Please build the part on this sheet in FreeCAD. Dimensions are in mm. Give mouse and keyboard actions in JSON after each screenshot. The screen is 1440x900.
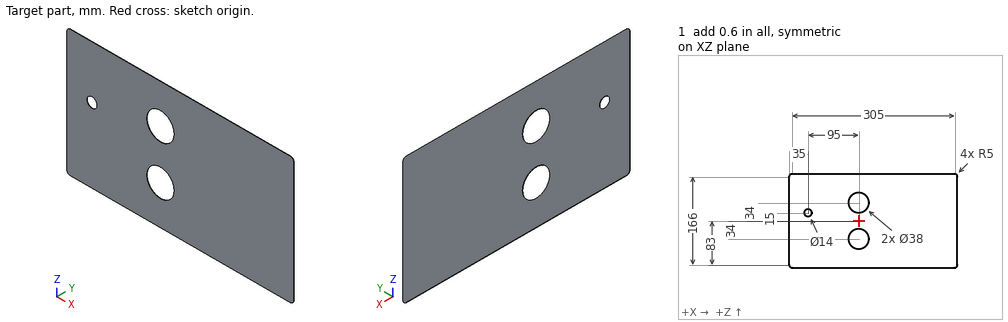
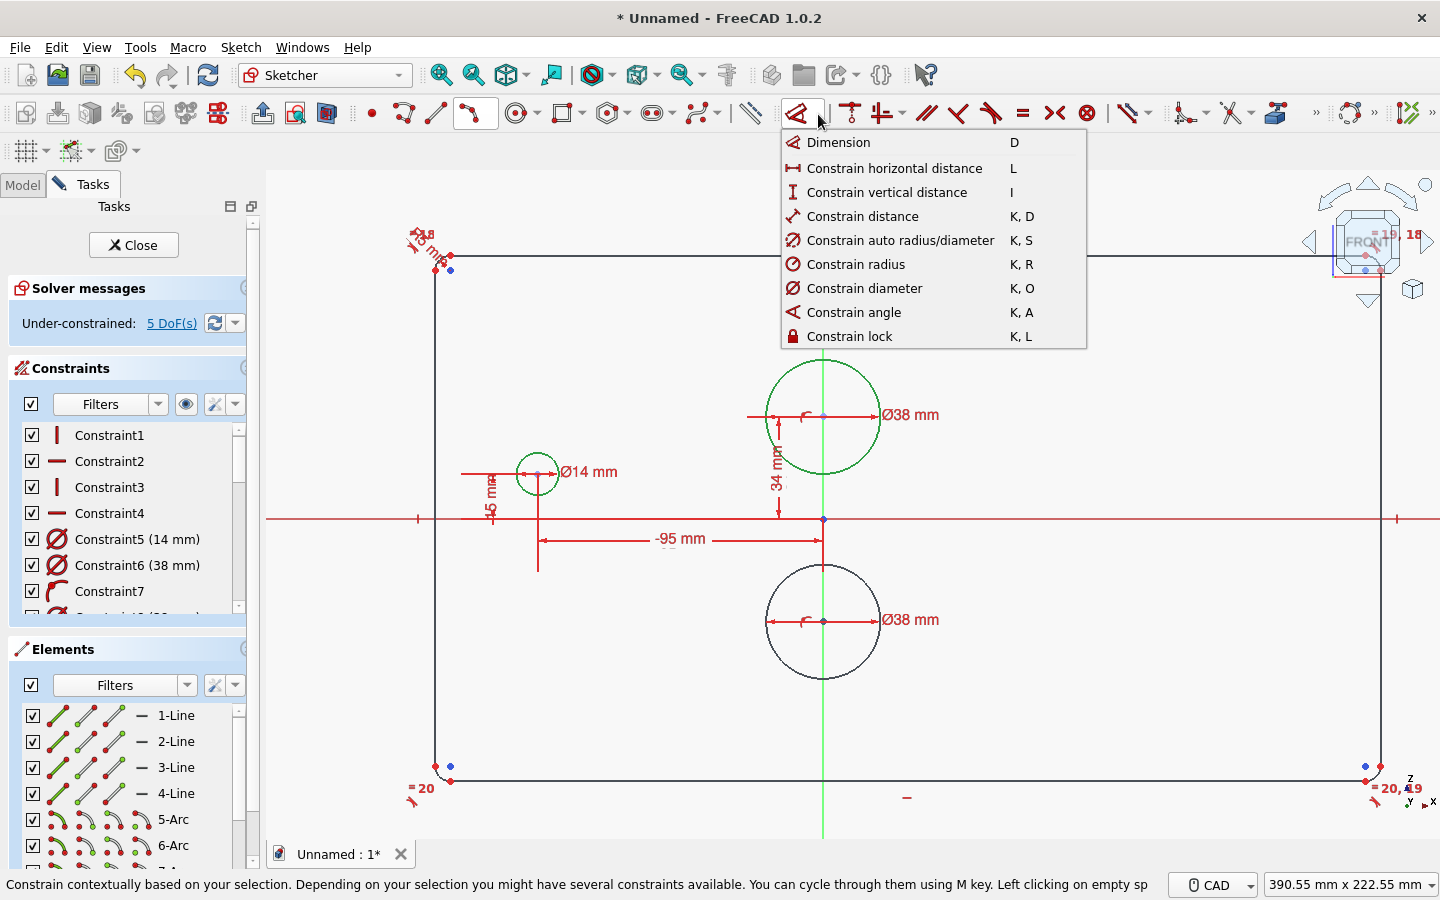
{"action": "left_click", "coordinate": [934, 192]}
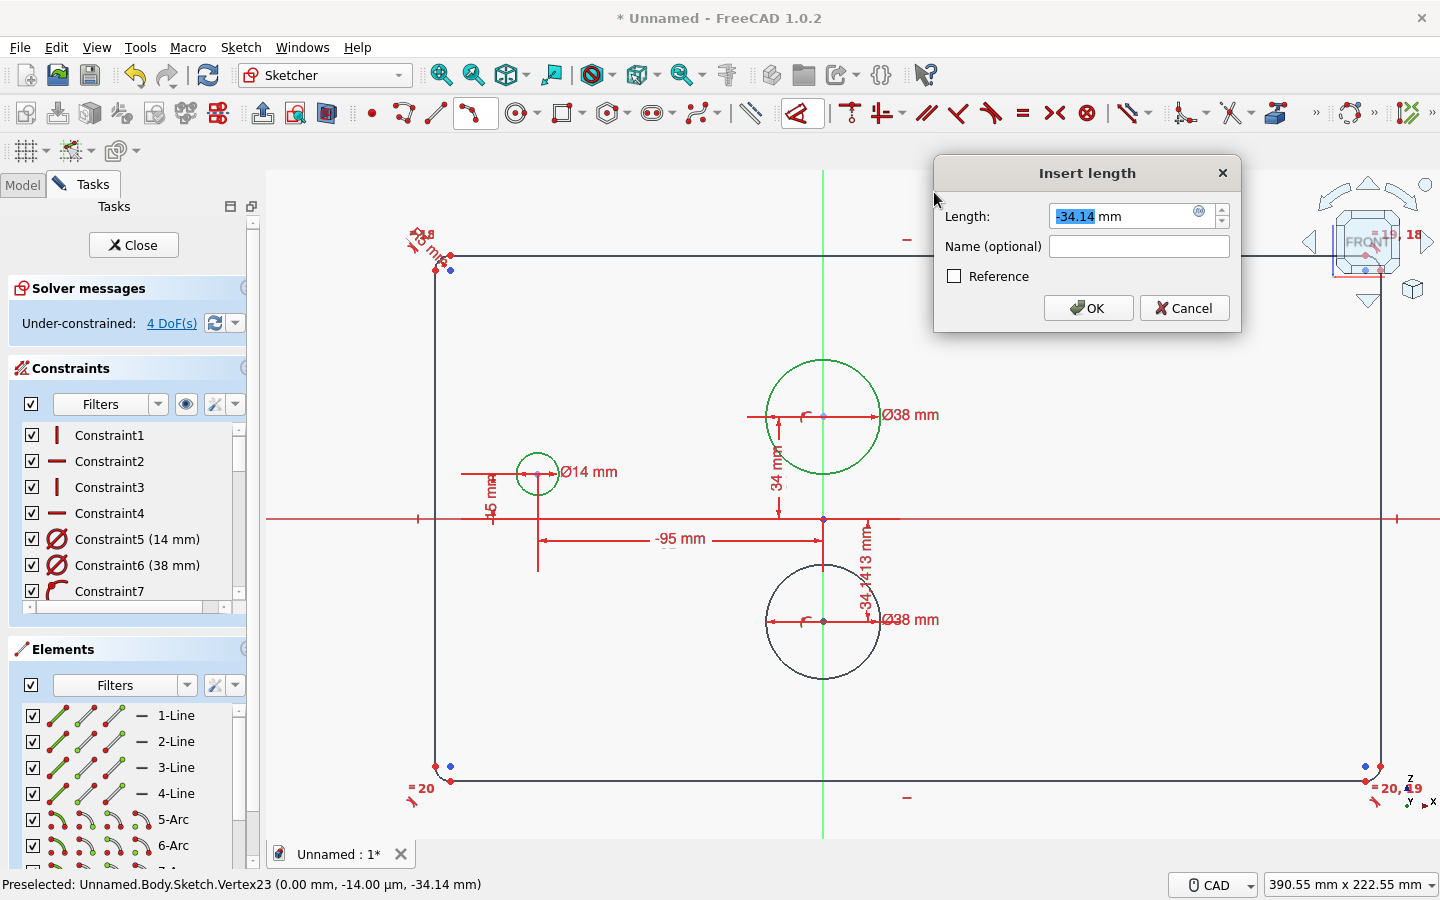
{"action": "type", "text": "-34"}
{"action": "key", "text": "Return"}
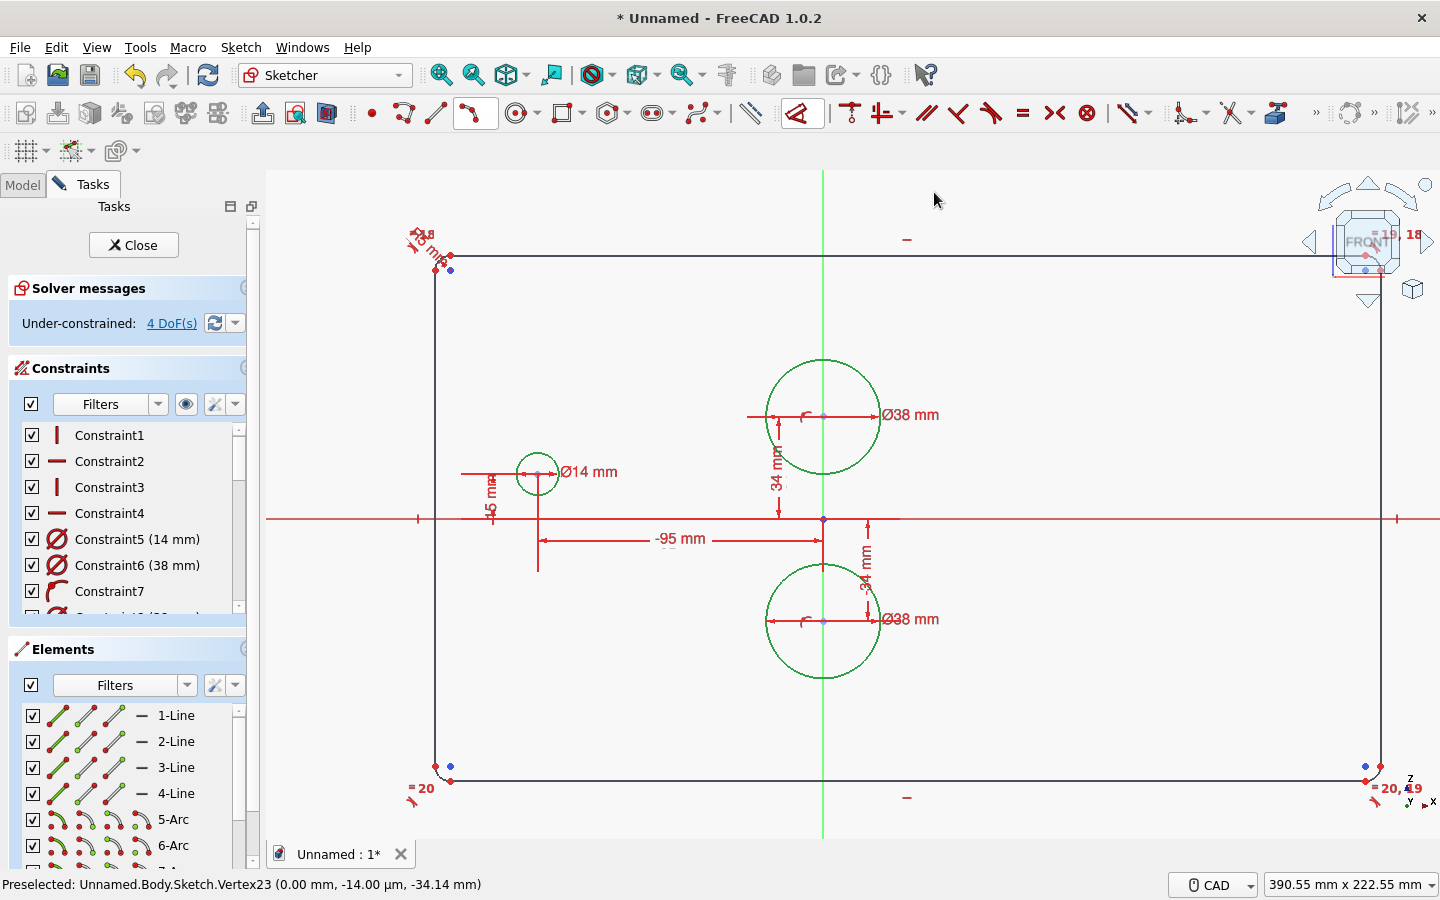
{"action": "left_click", "coordinate": [435, 617]}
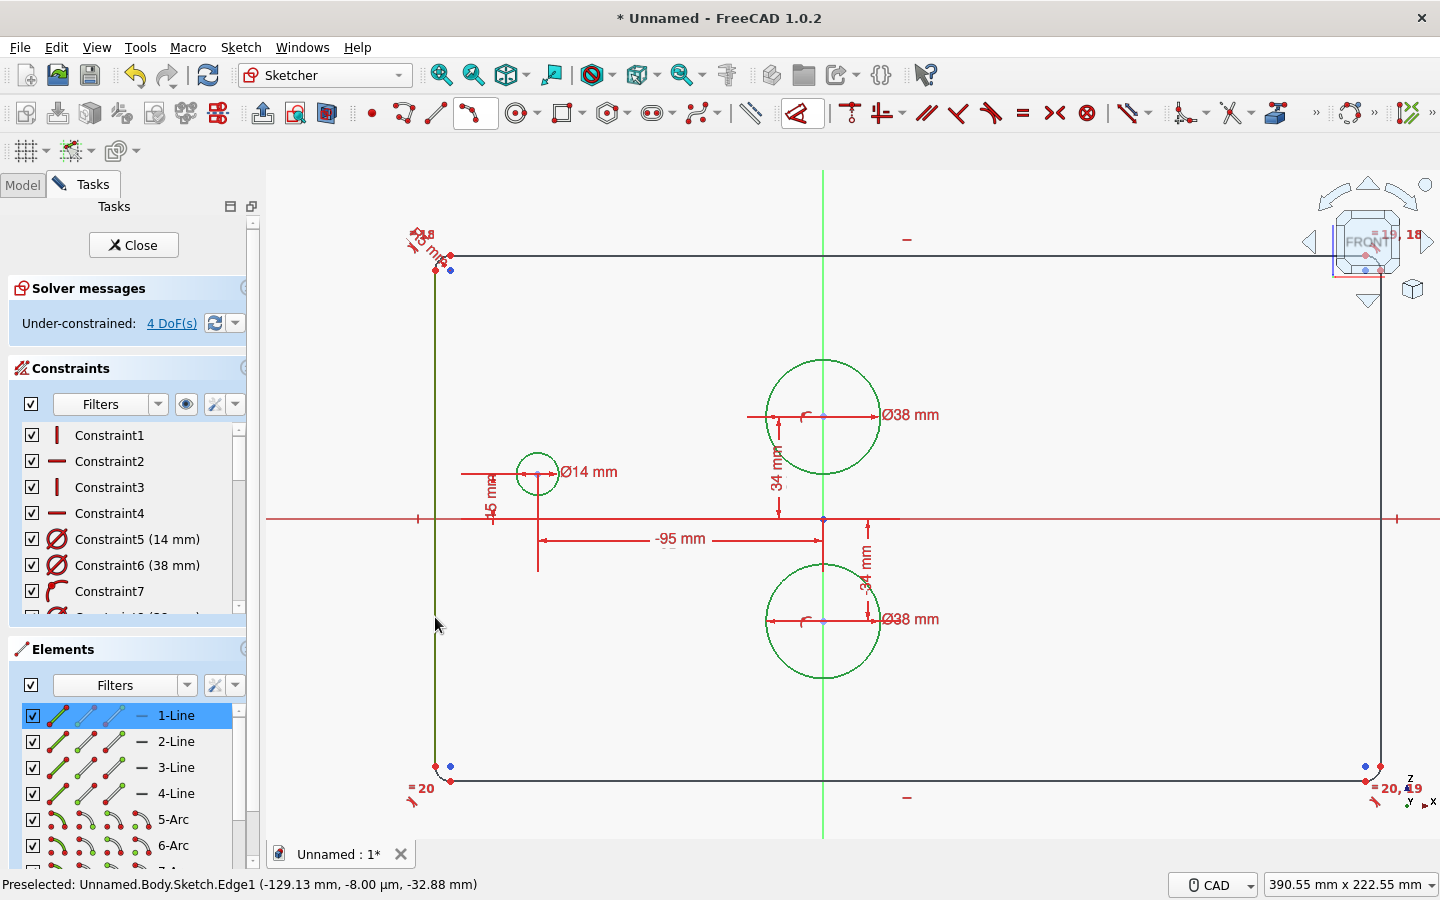
{"action": "left_click", "coordinate": [818, 114]}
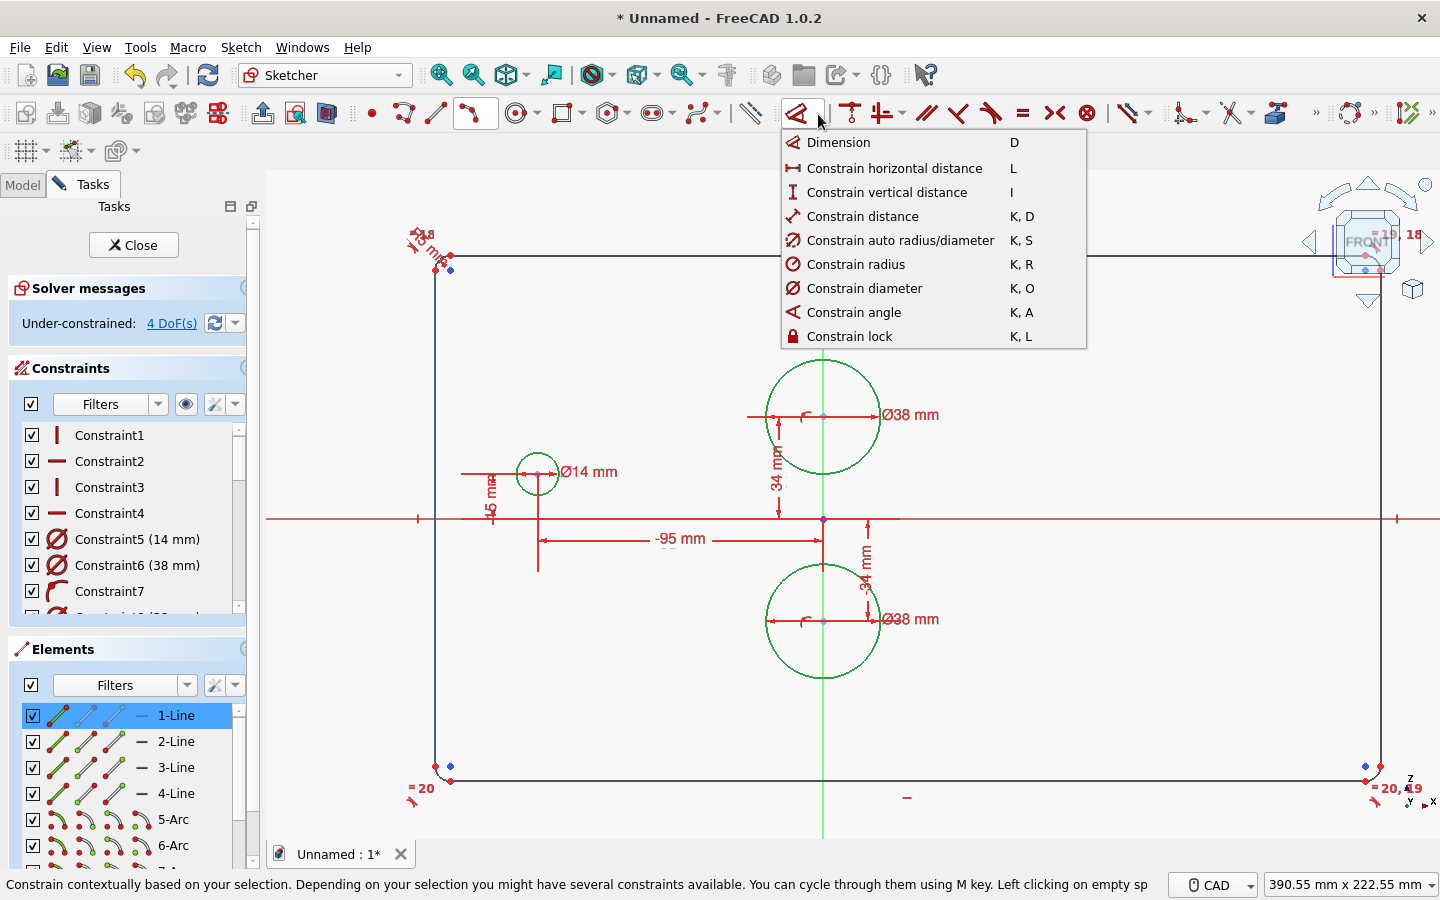
{"action": "left_click", "coordinate": [934, 192]}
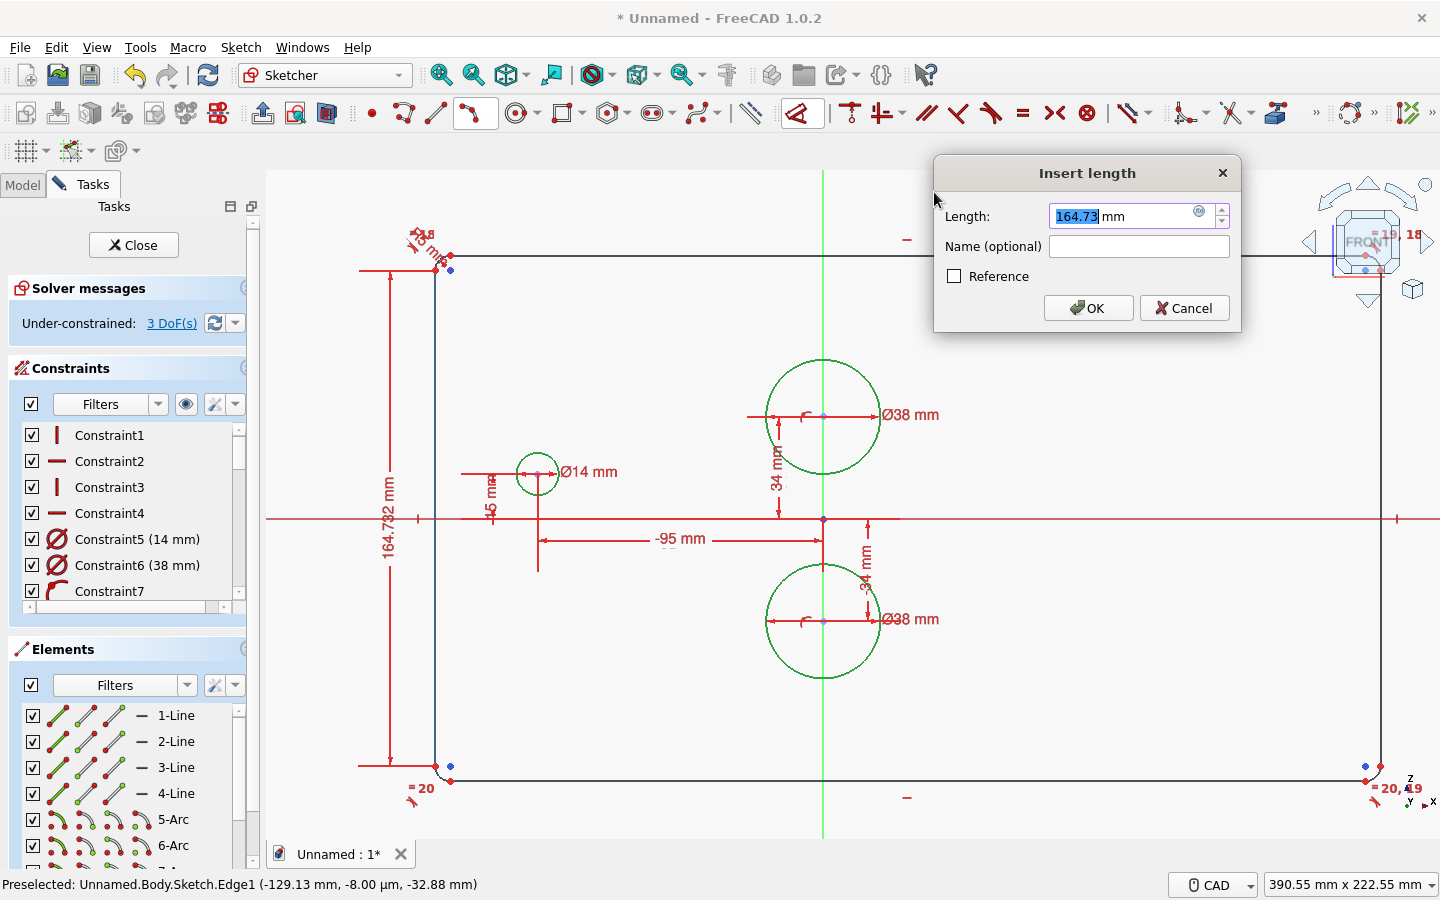
{"action": "type", "text": "166"}
{"action": "key", "text": "Return"}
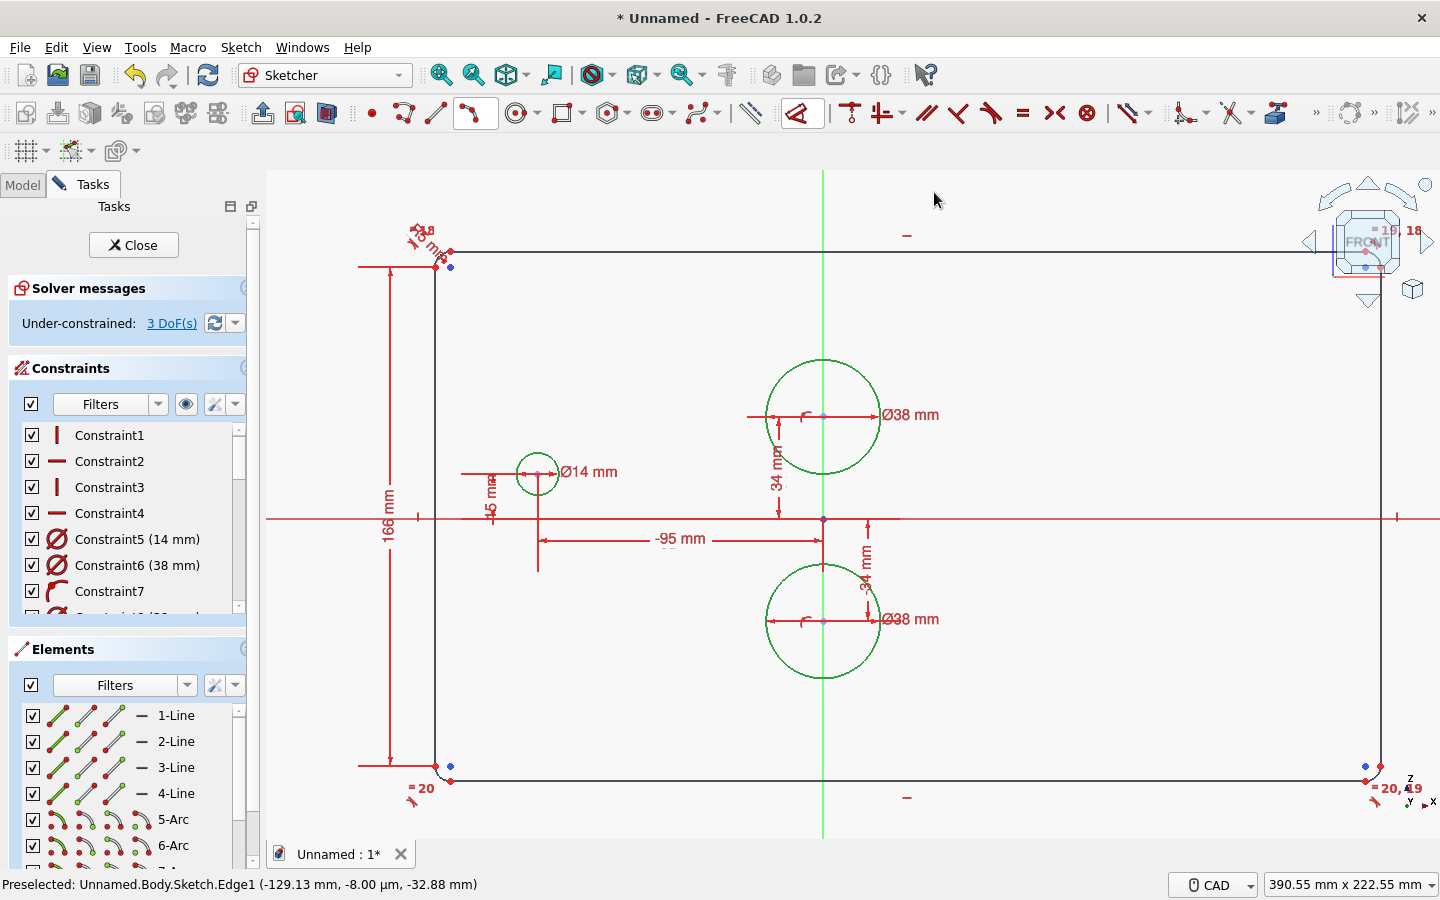
{"action": "left_click", "coordinate": [725, 252]}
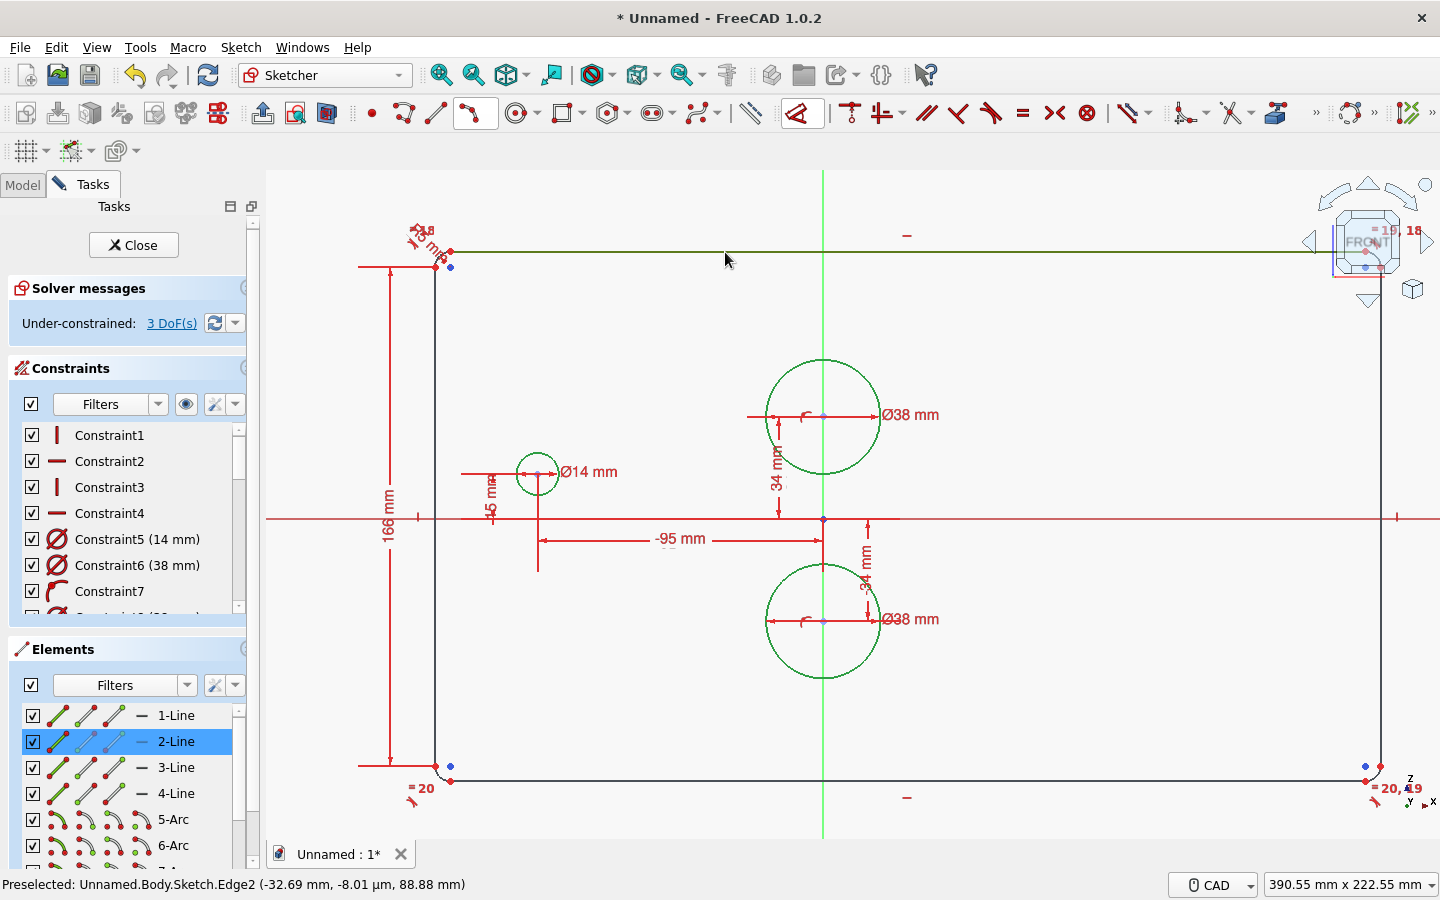
{"action": "key", "text": "l"}